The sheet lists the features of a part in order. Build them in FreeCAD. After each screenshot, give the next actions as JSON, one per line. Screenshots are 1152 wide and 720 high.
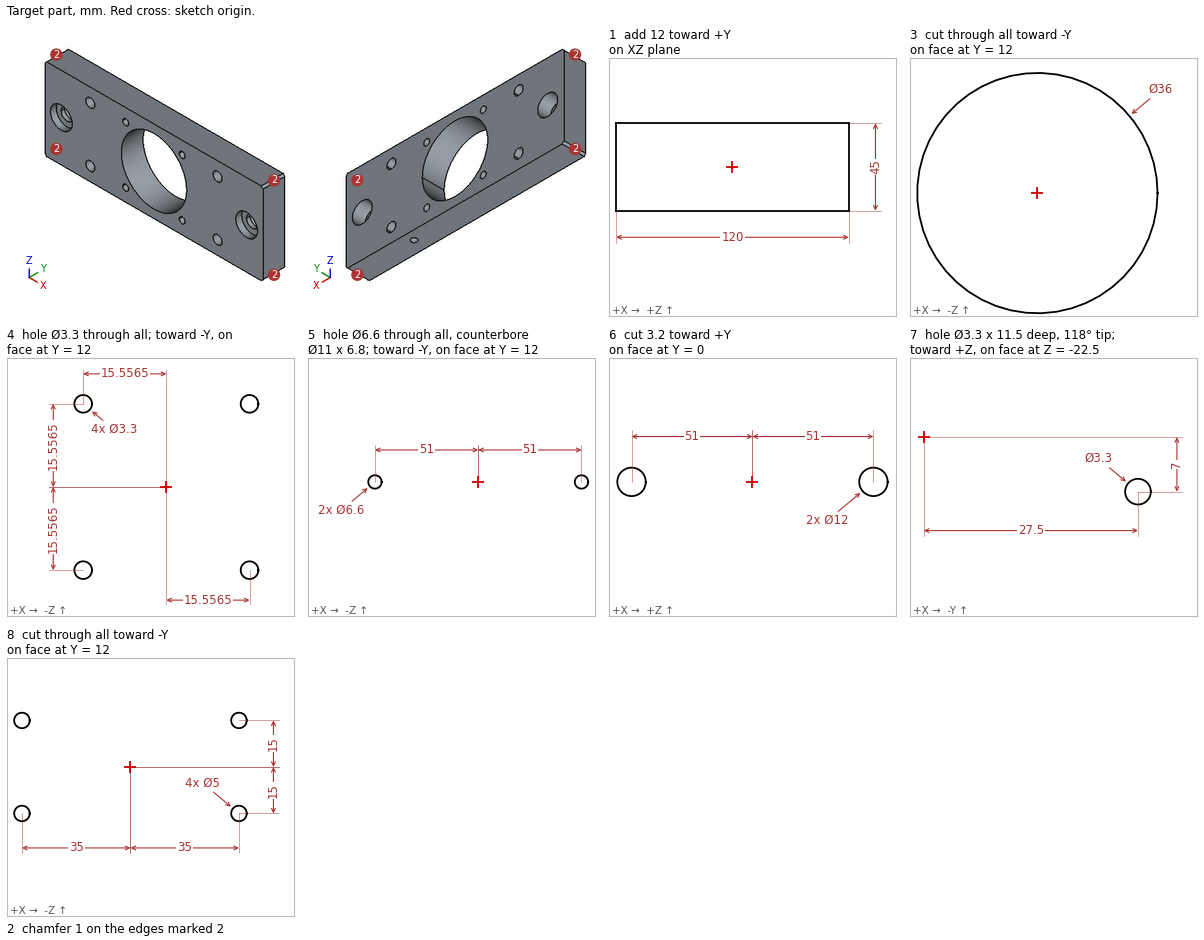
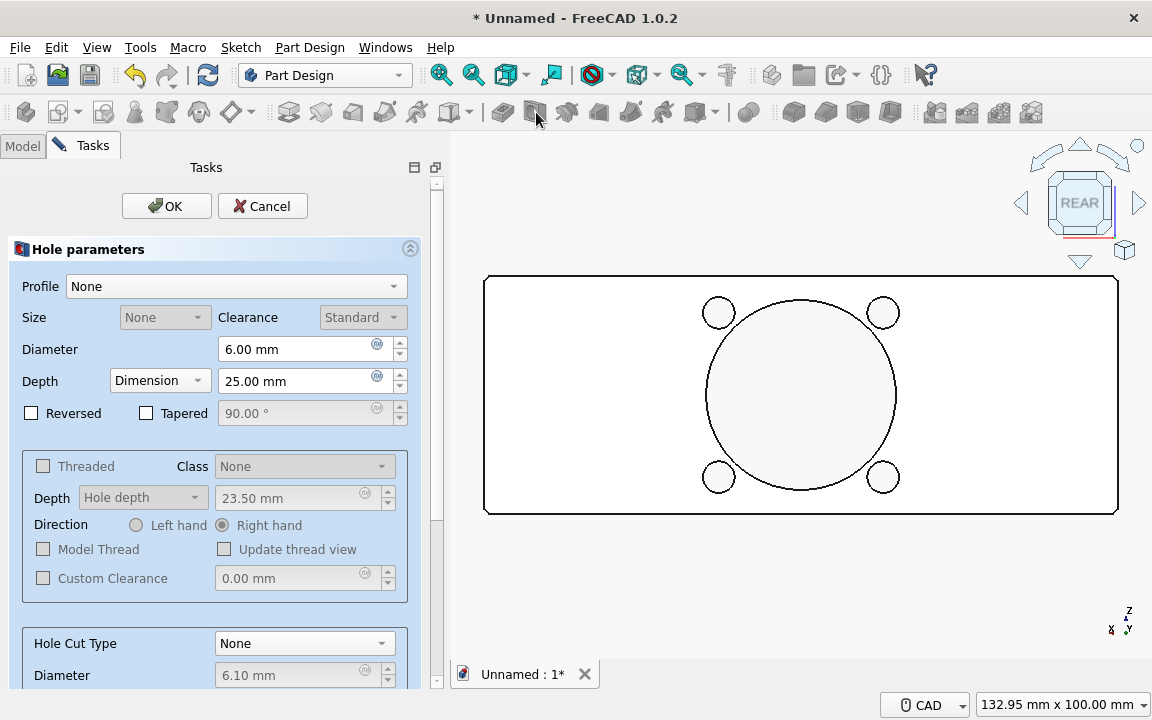
{"action": "triple_click", "coordinate": [305, 349]}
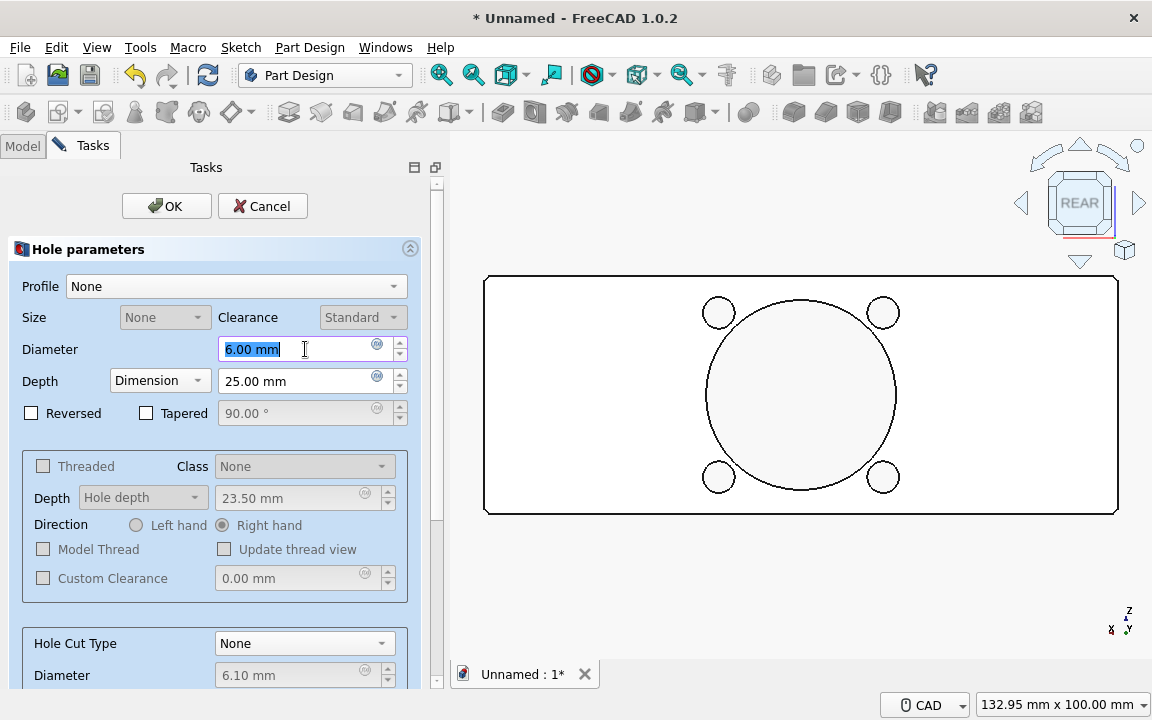
{"action": "type", "text": "3.3"}
{"action": "key", "text": "Tab"}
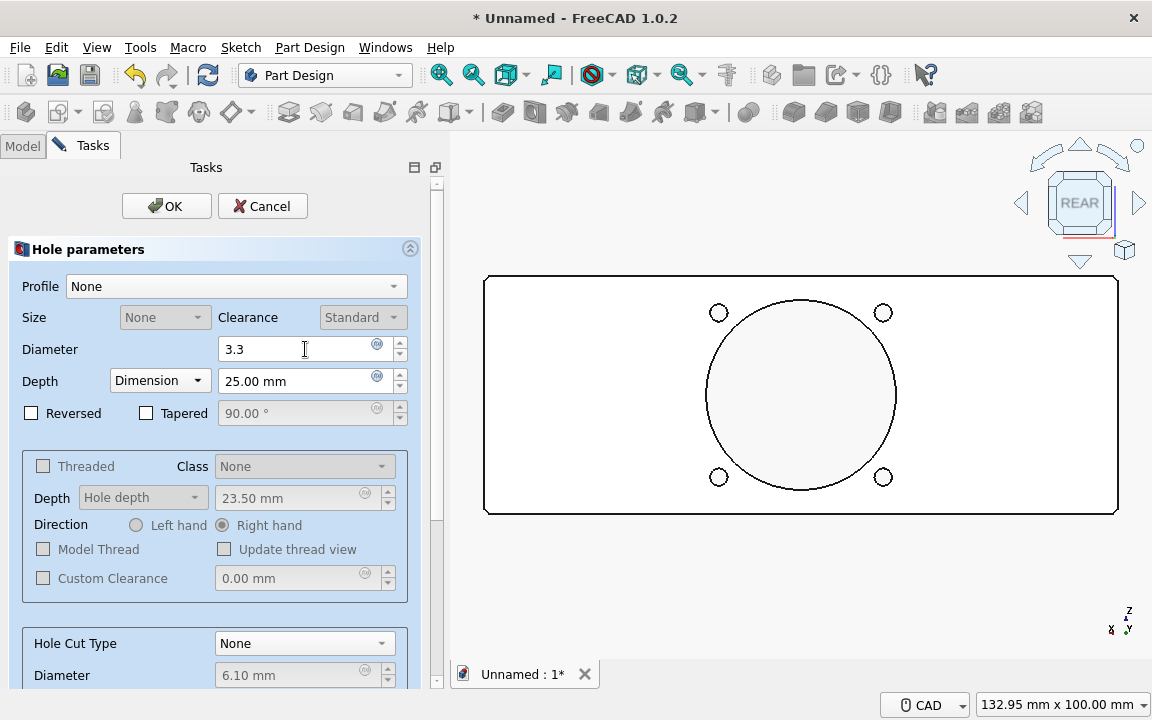
{"action": "left_click", "coordinate": [161, 380]}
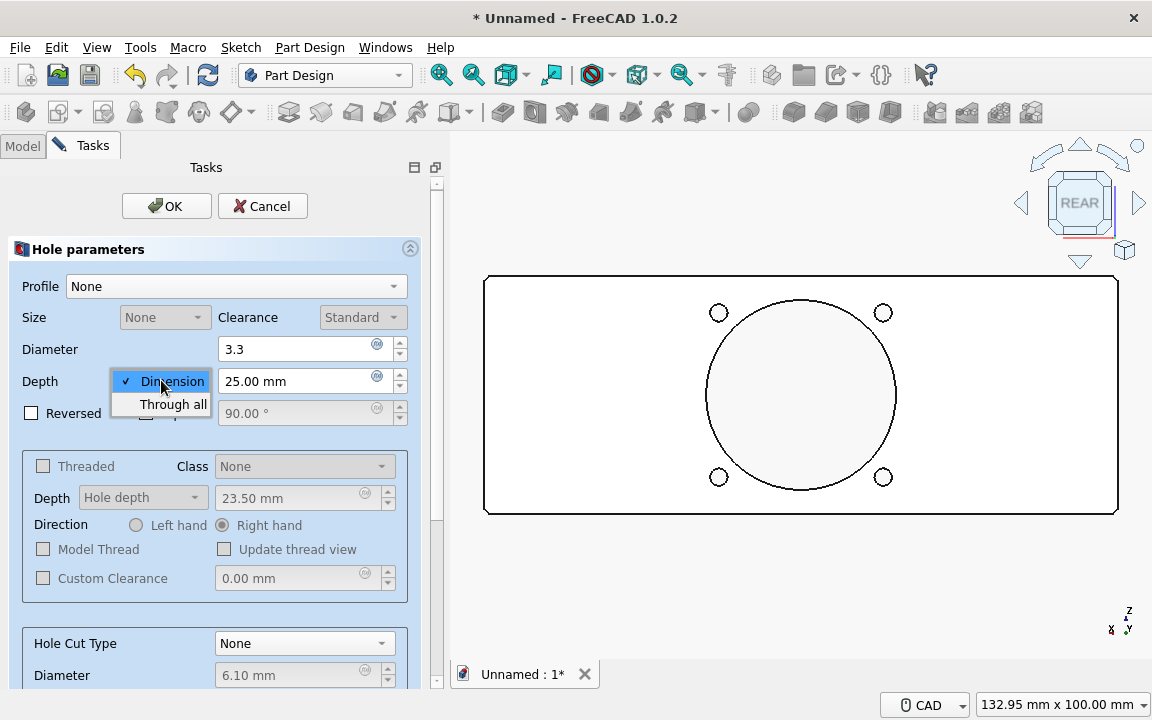
{"action": "left_click", "coordinate": [160, 404]}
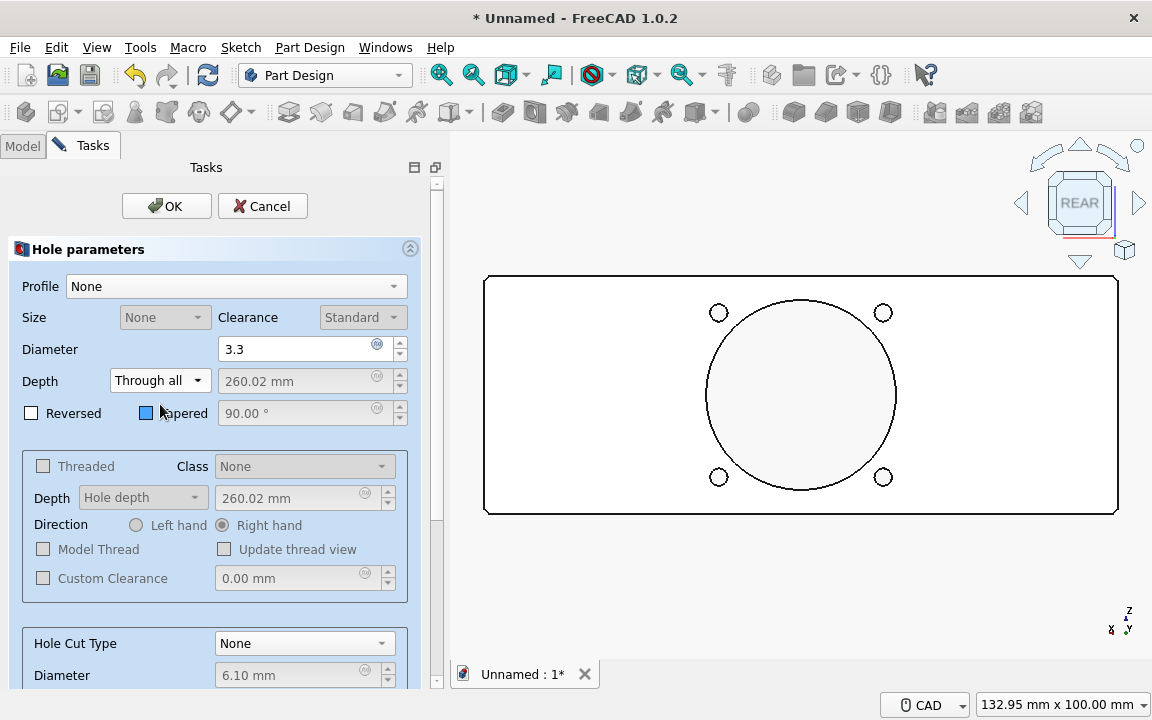
{"action": "left_click", "coordinate": [167, 206]}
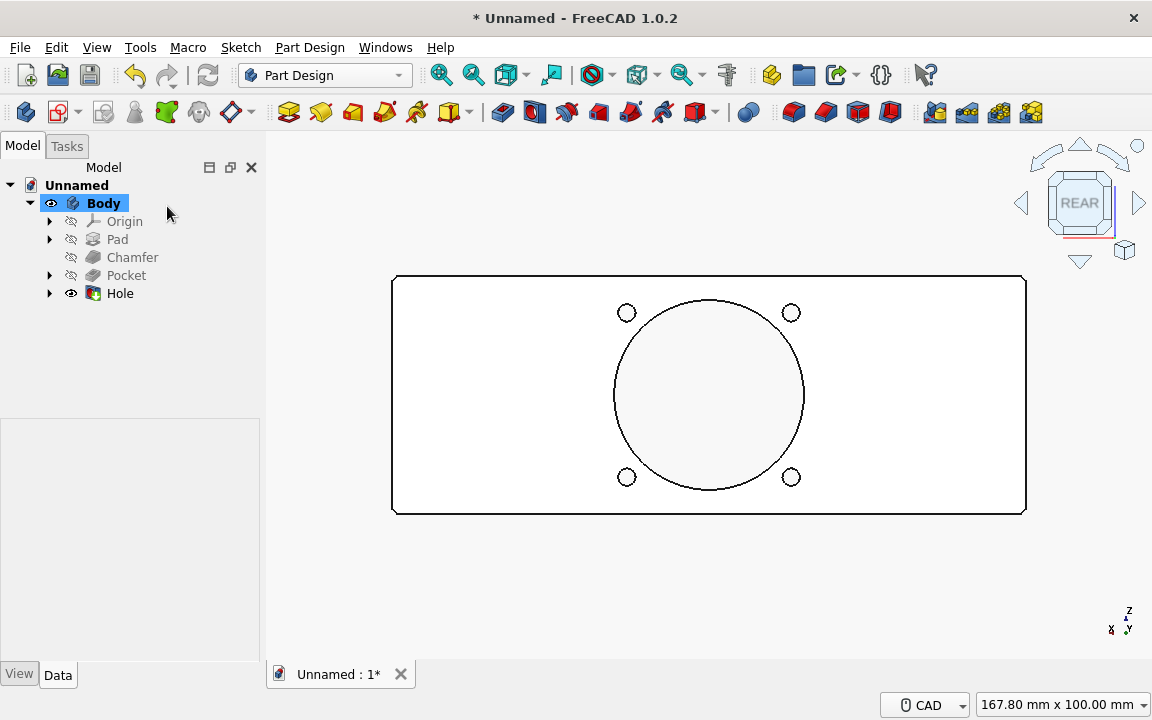
{"action": "left_click", "coordinate": [528, 394]}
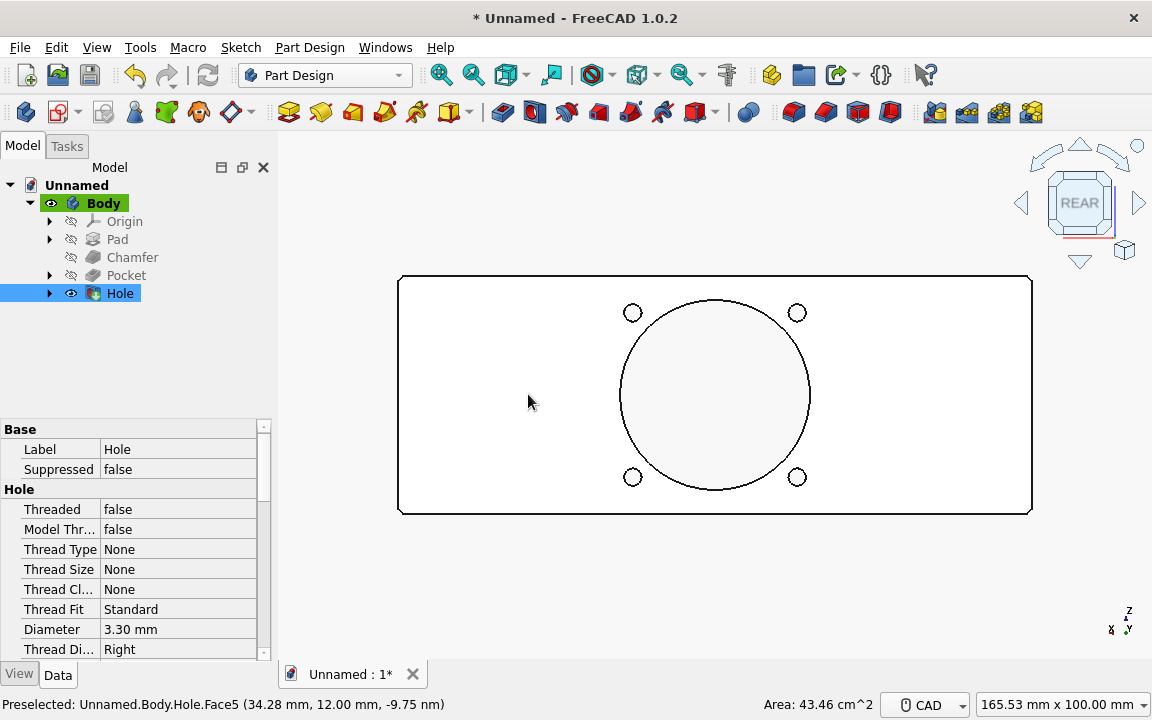
{"action": "left_click", "coordinate": [58, 112]}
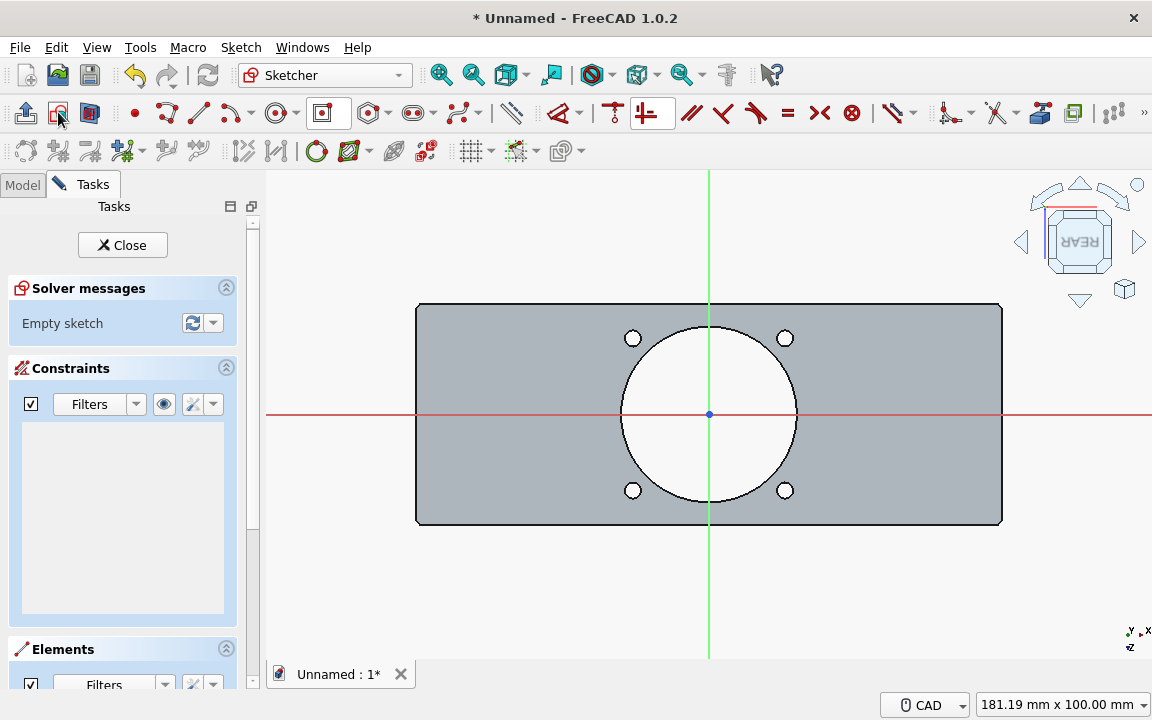
{"action": "scroll", "coordinate": [331, 415], "scroll_direction": "down", "scroll_amount": 1}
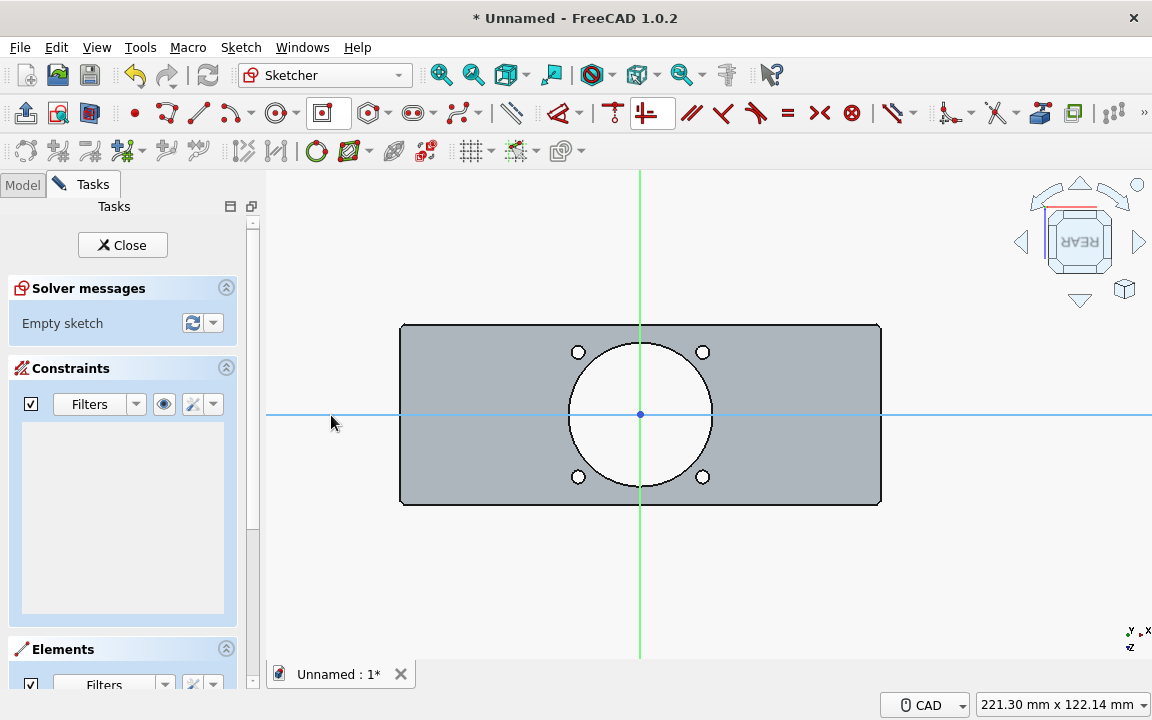
{"action": "left_click", "coordinate": [276, 114]}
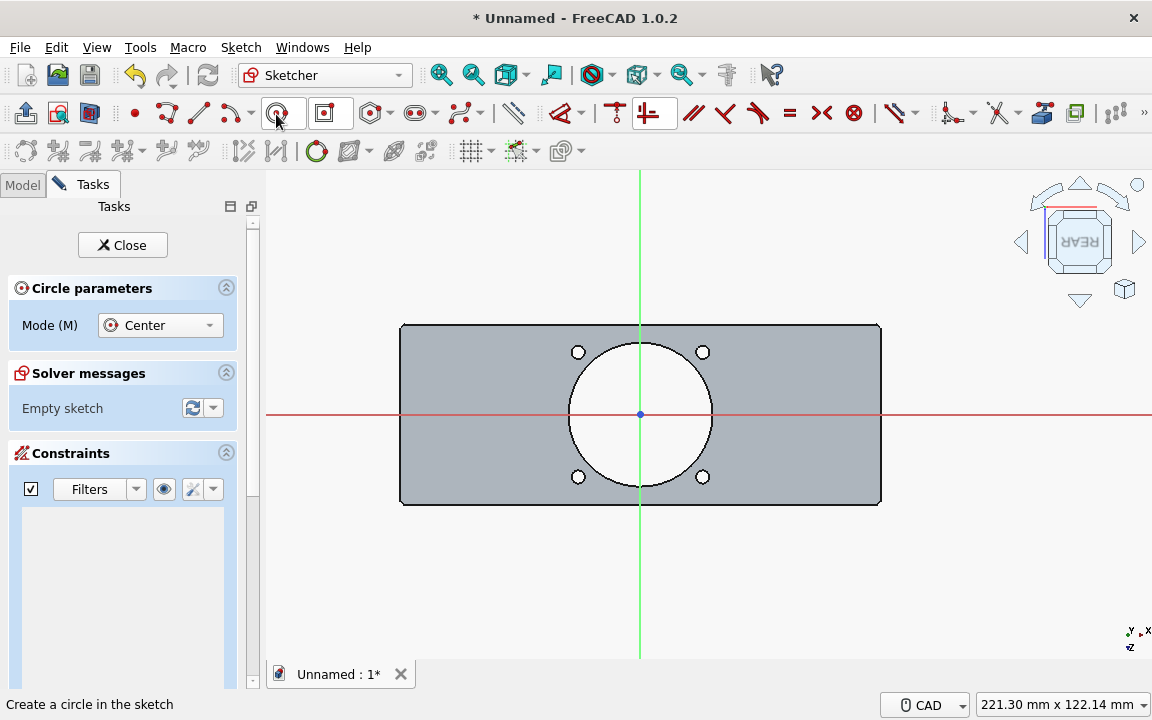
{"action": "scroll", "coordinate": [436, 415], "scroll_direction": "up", "scroll_amount": 3}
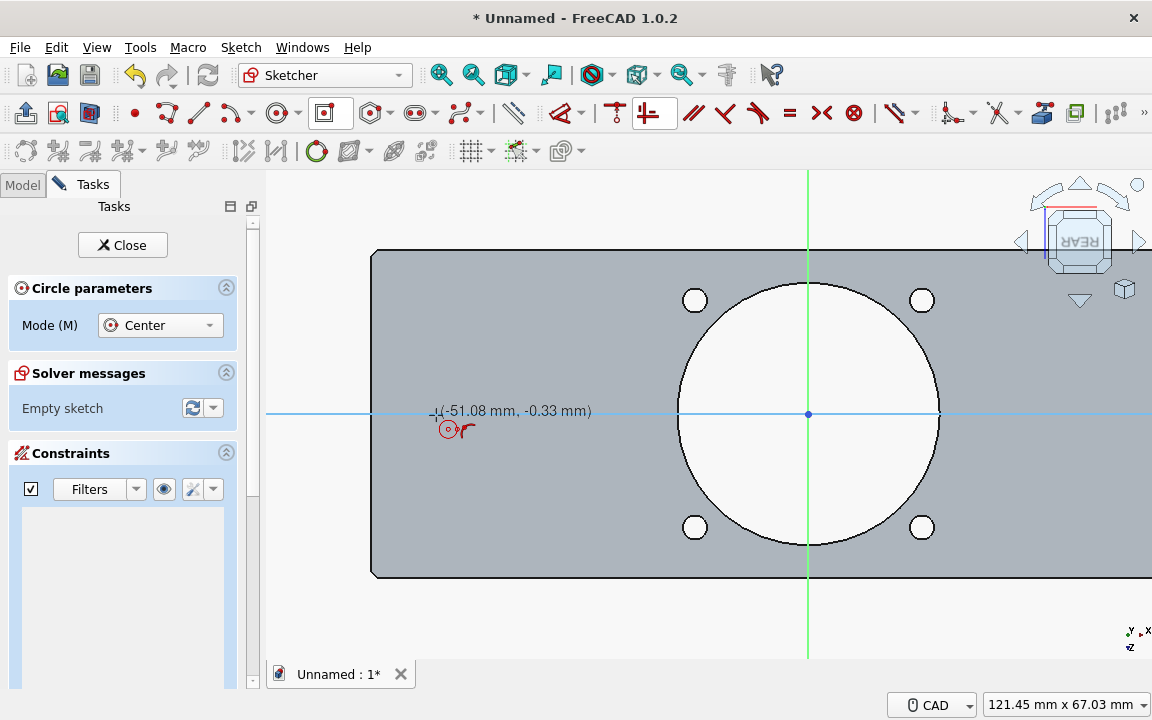
{"action": "left_click", "coordinate": [436, 414]}
{"action": "mouse_move", "coordinate": [453, 397]}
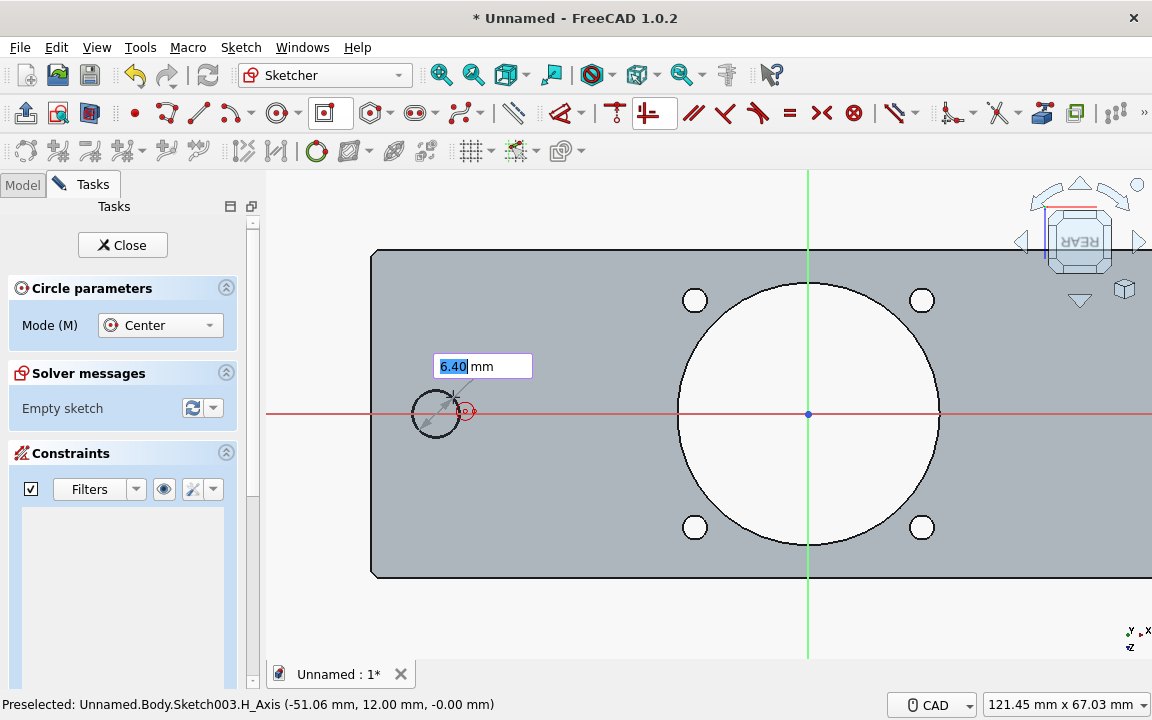
{"action": "type", "text": "6.6"}
{"action": "key", "text": "Return"}